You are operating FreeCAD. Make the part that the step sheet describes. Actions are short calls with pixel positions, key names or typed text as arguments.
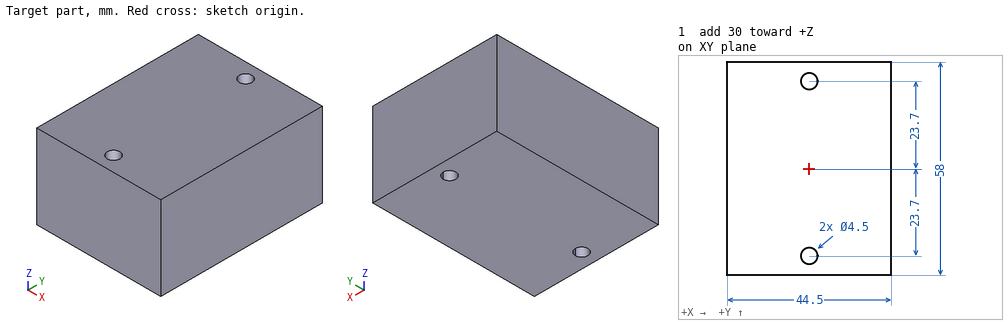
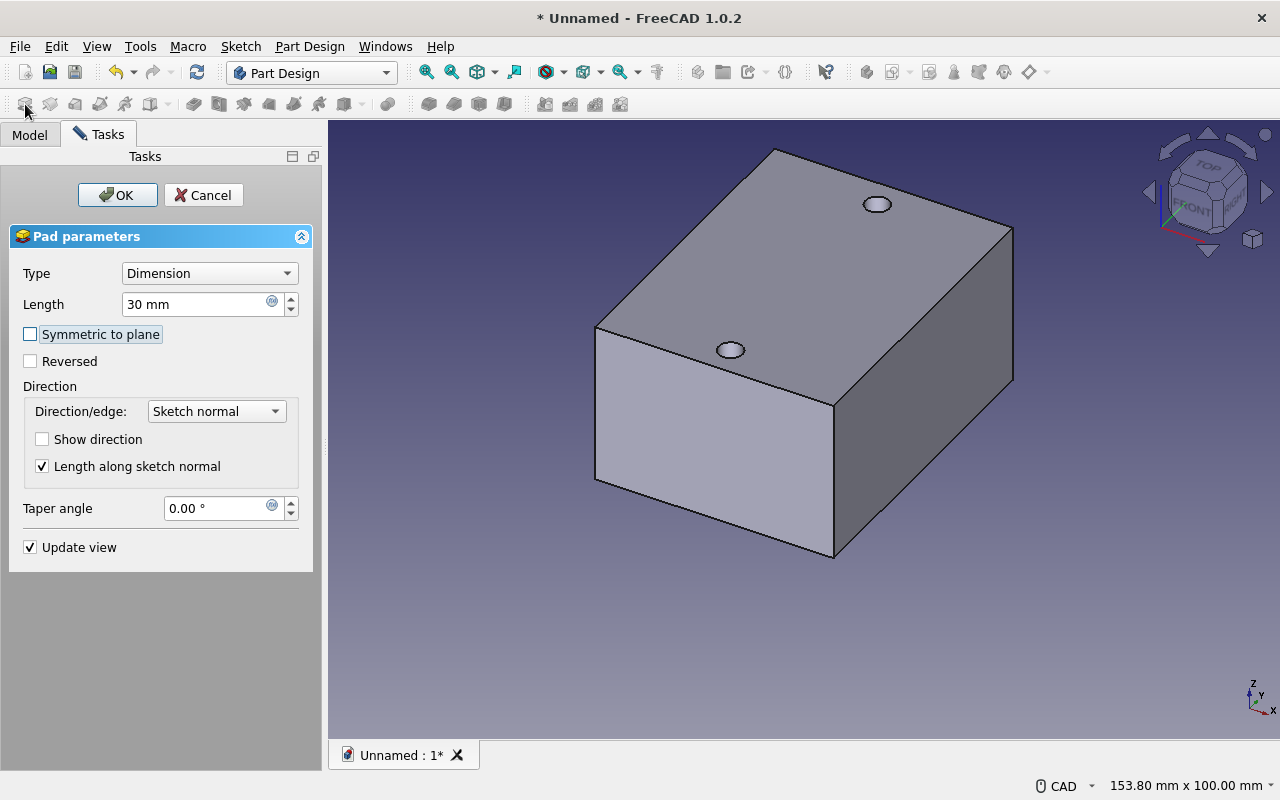
click(118, 195)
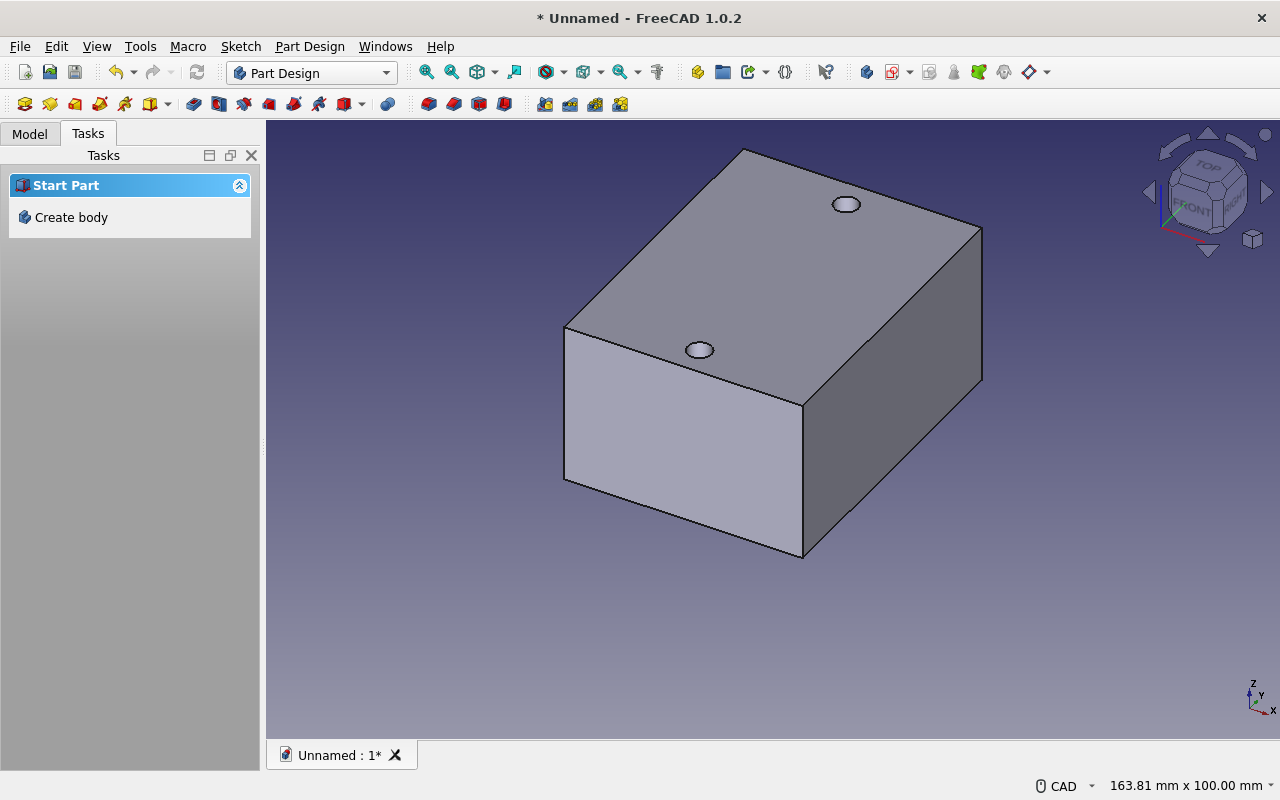
key(0)